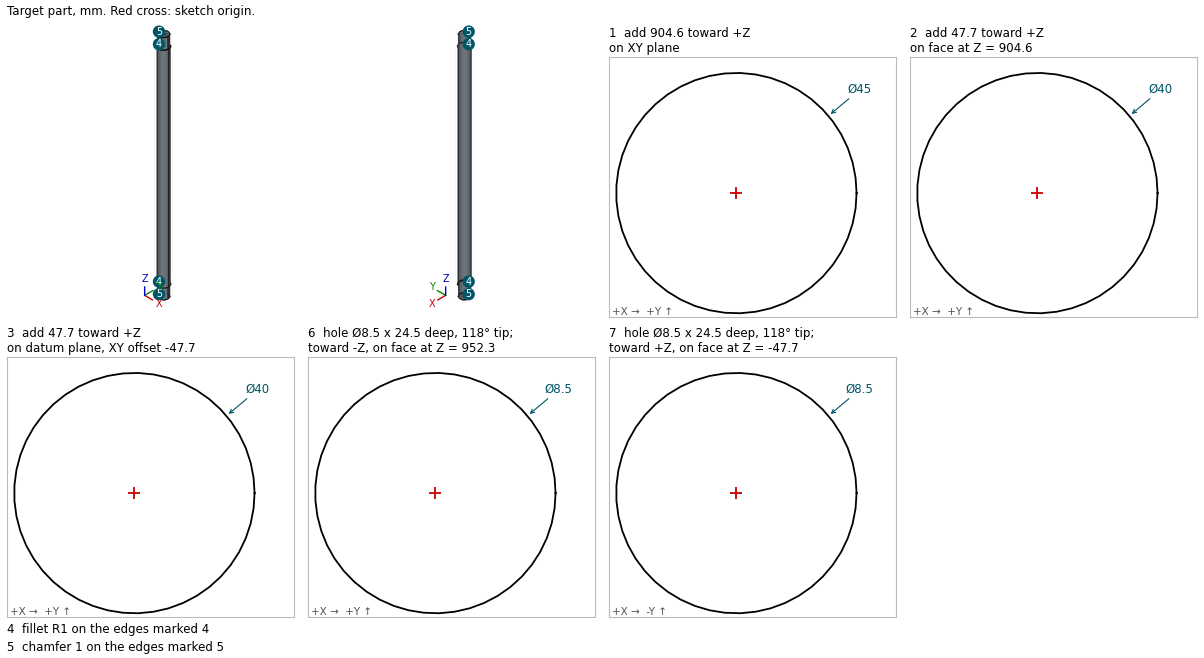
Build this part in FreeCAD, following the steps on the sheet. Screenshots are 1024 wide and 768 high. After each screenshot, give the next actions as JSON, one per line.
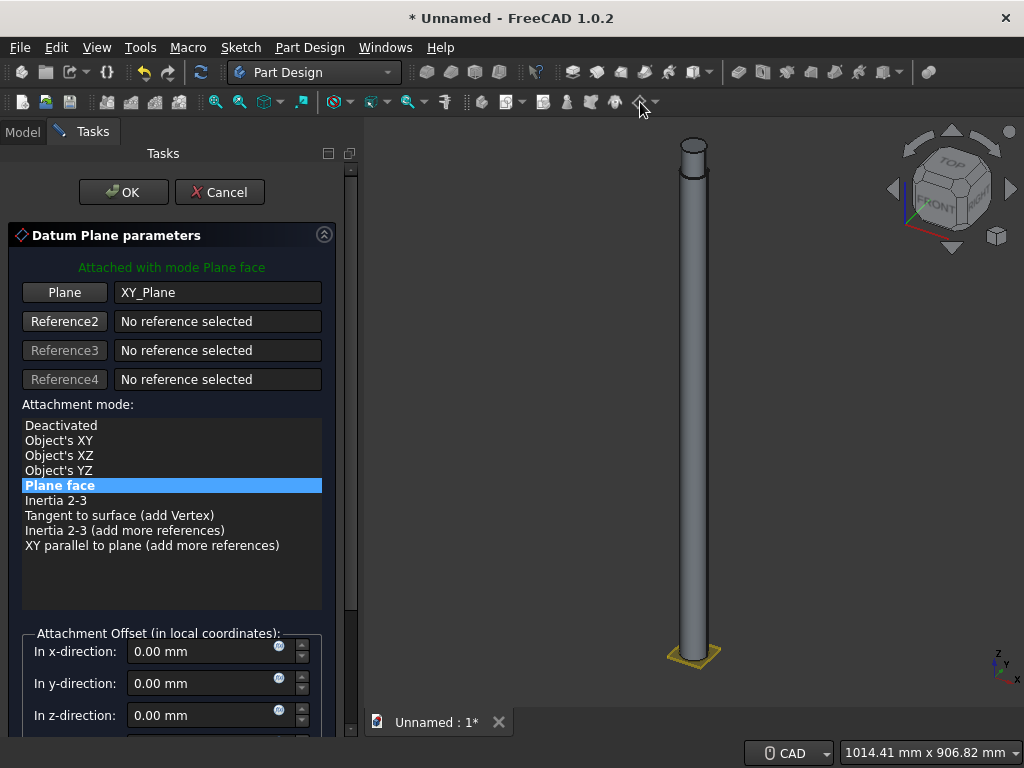
{"action": "triple_click", "coordinate": [210, 715]}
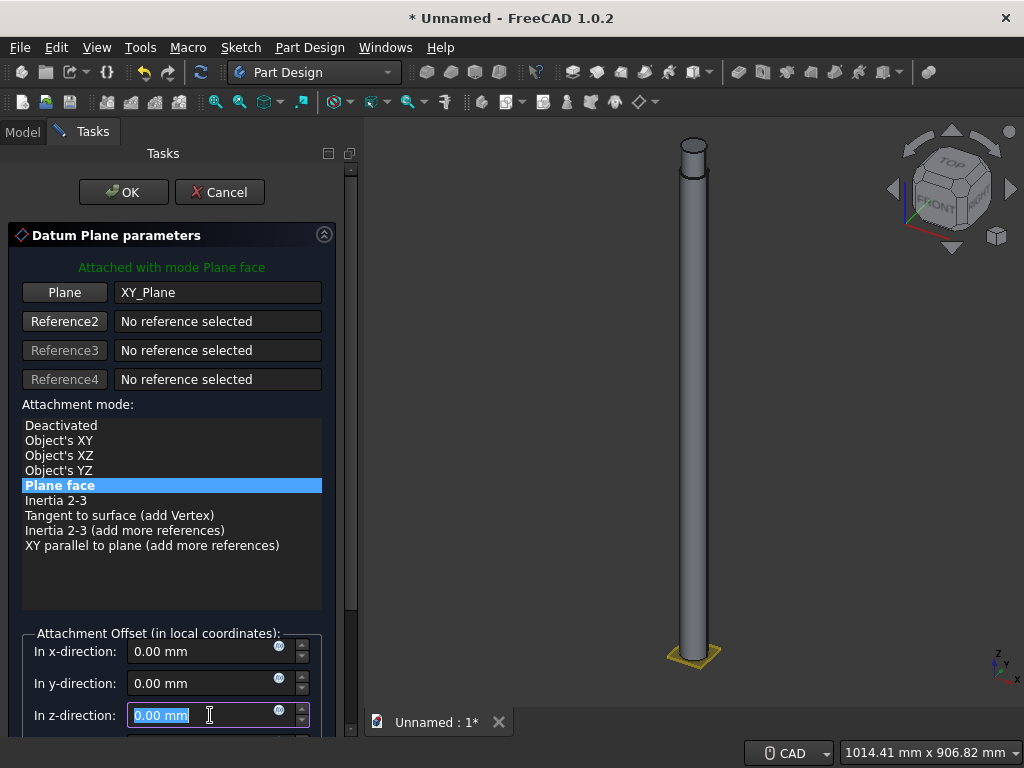
{"action": "type", "text": "-47.7"}
{"action": "key", "text": "Tab"}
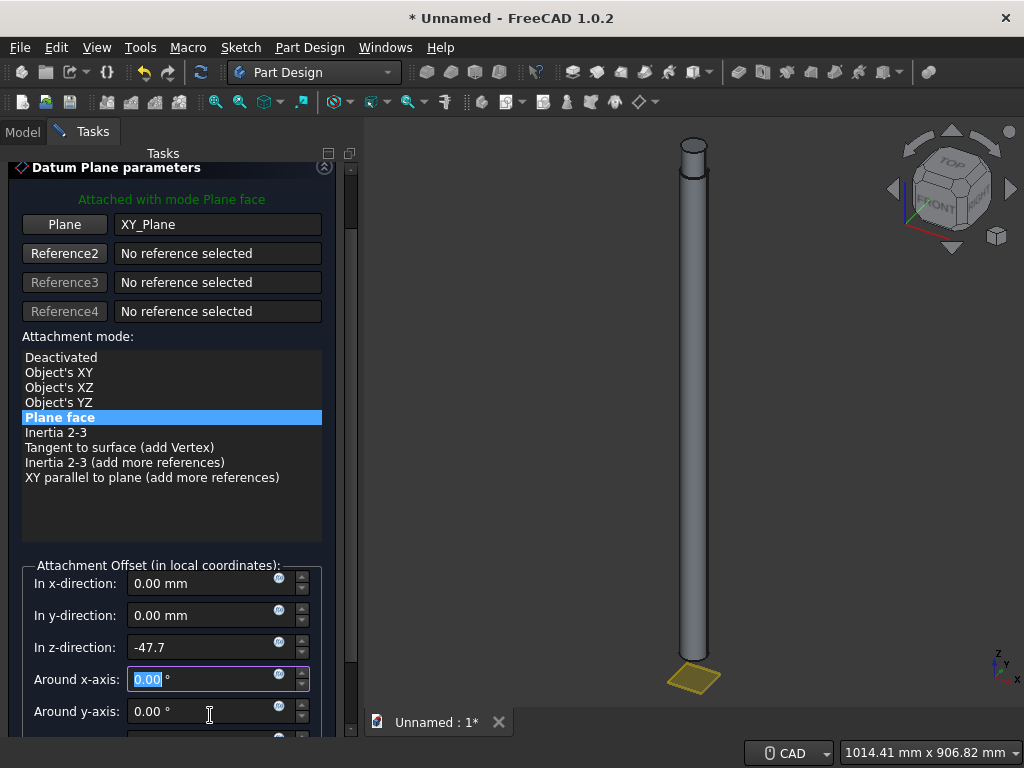
{"action": "scroll", "coordinate": [351, 450], "scroll_direction": "up", "scroll_amount": 2}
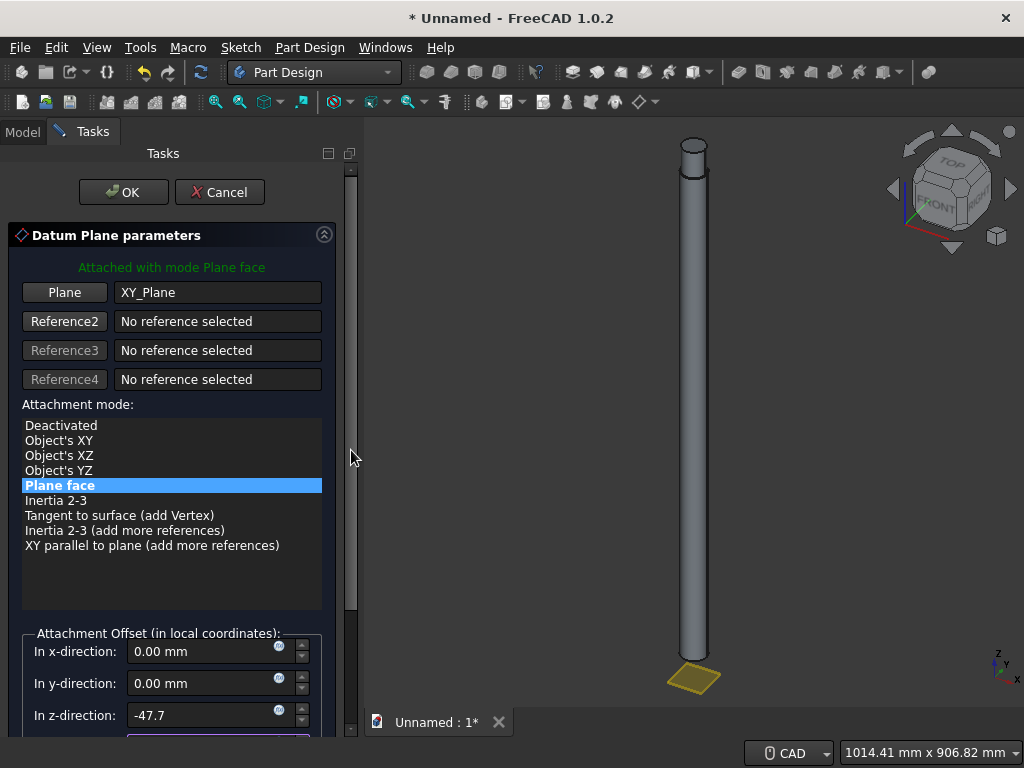
{"action": "left_click", "coordinate": [124, 192]}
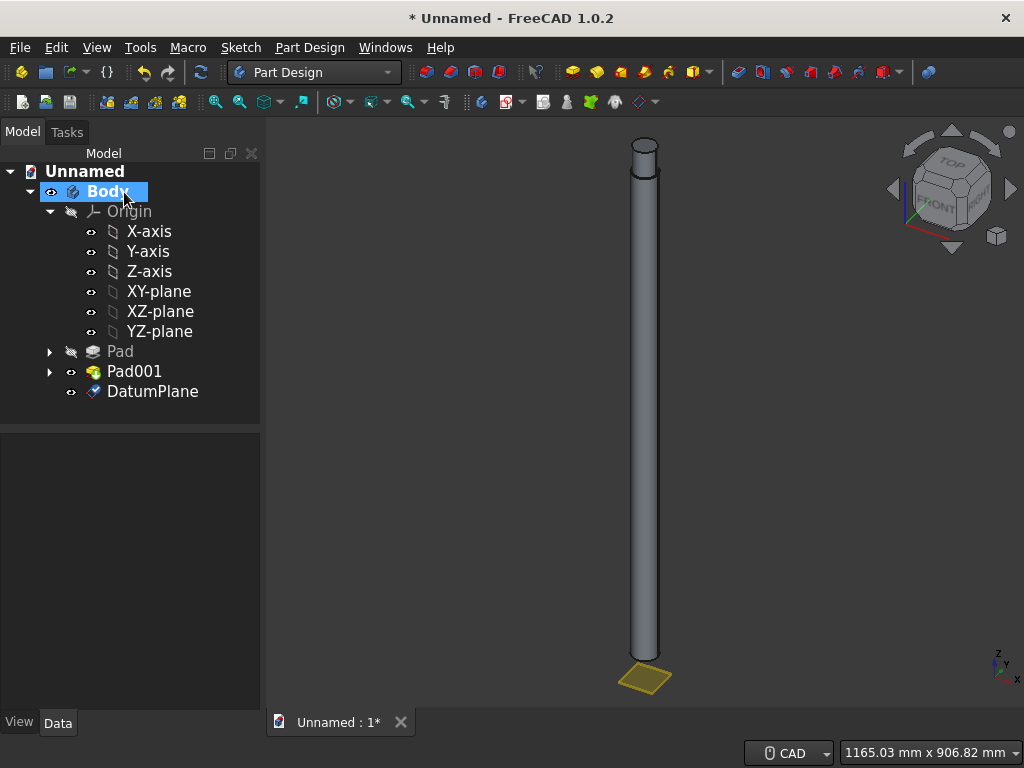
{"action": "left_click", "coordinate": [116, 392]}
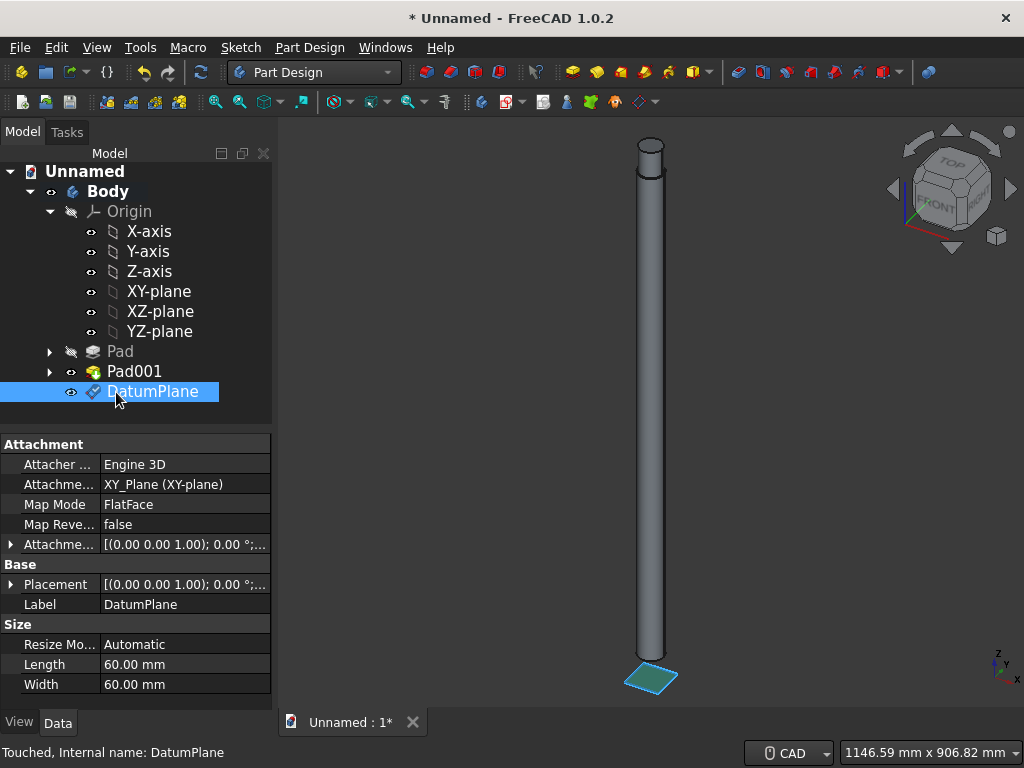
{"action": "left_click", "coordinate": [506, 102]}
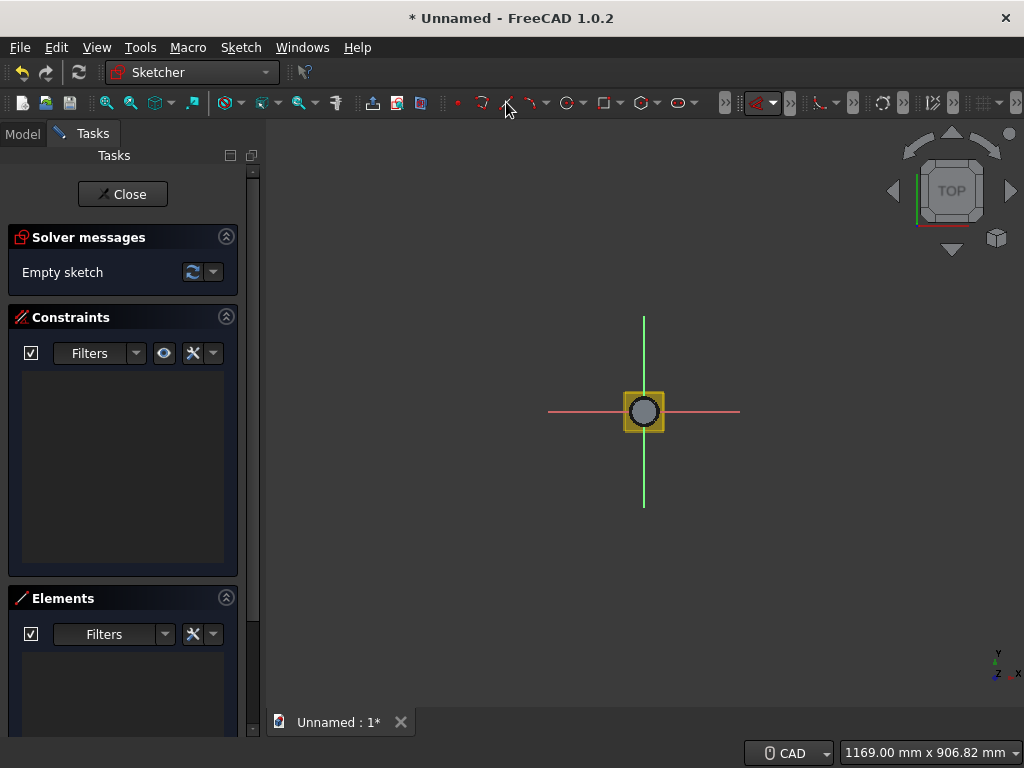
{"action": "left_click", "coordinate": [422, 104]}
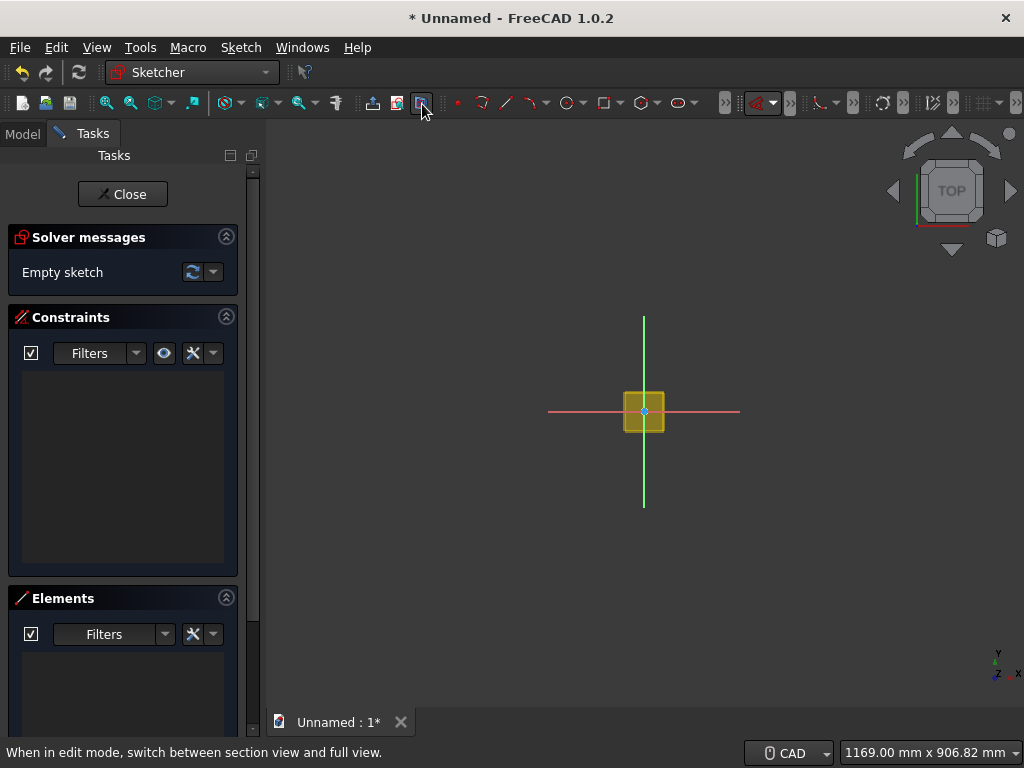
{"action": "scroll", "coordinate": [650, 412], "scroll_direction": "up", "scroll_amount": 13}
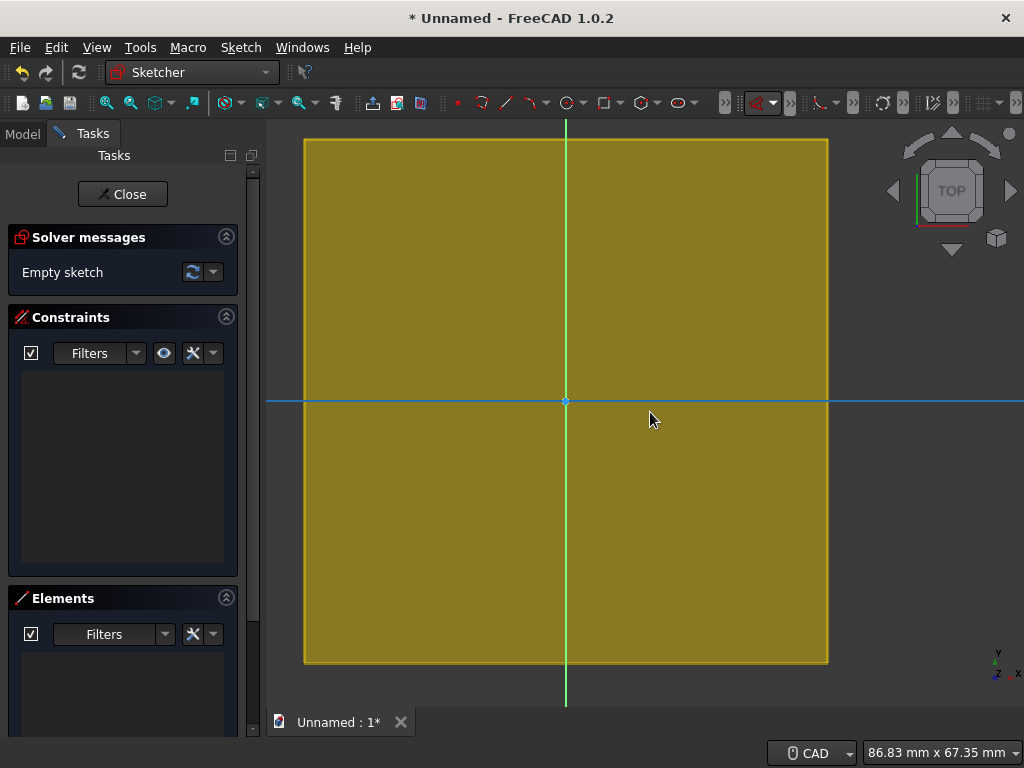
{"action": "left_click", "coordinate": [568, 104]}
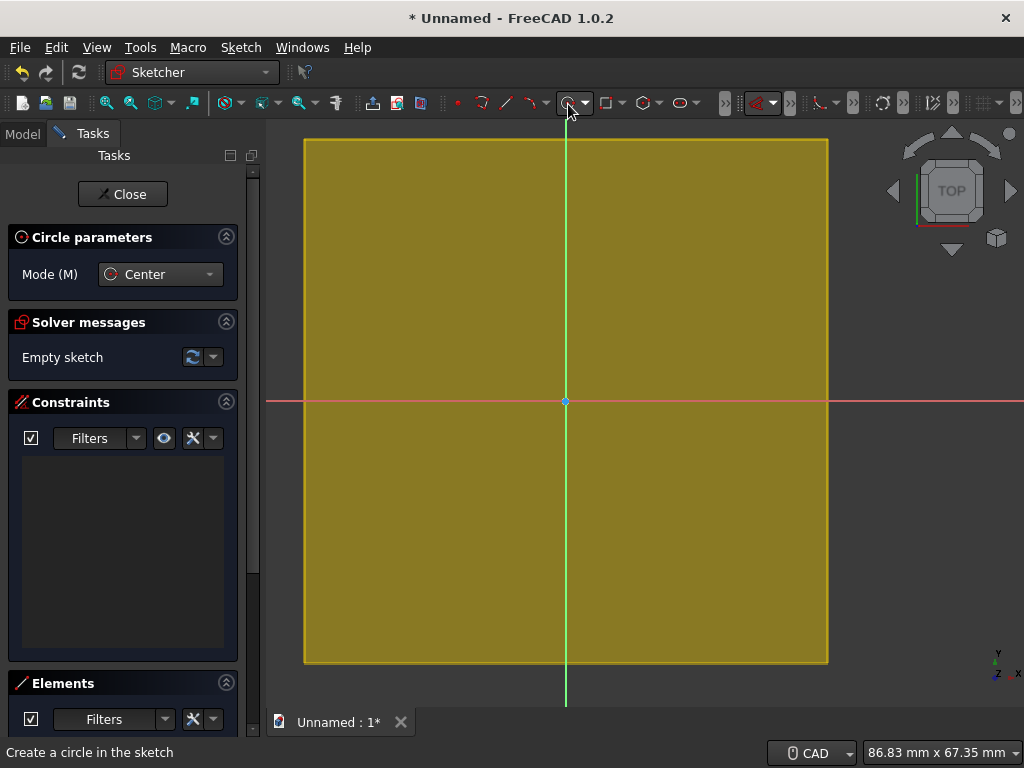
{"action": "left_click", "coordinate": [566, 401]}
{"action": "mouse_move", "coordinate": [689, 278]}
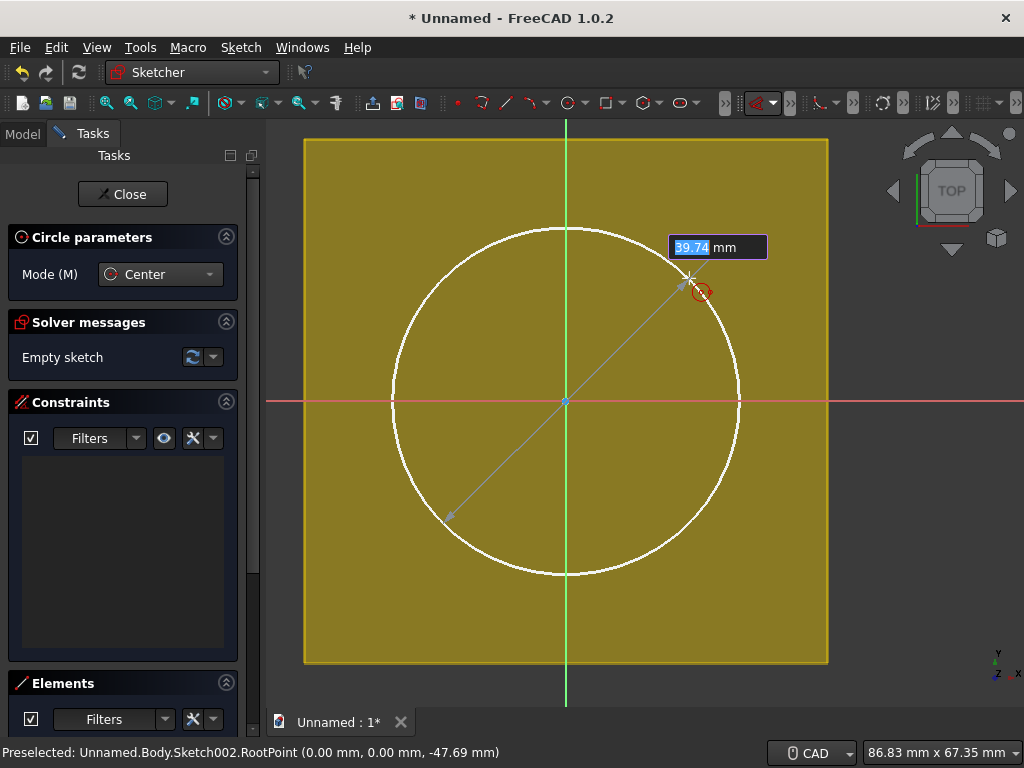
{"action": "type", "text": "40"}
{"action": "key", "text": "Return"}
{"action": "key", "text": "Escape"}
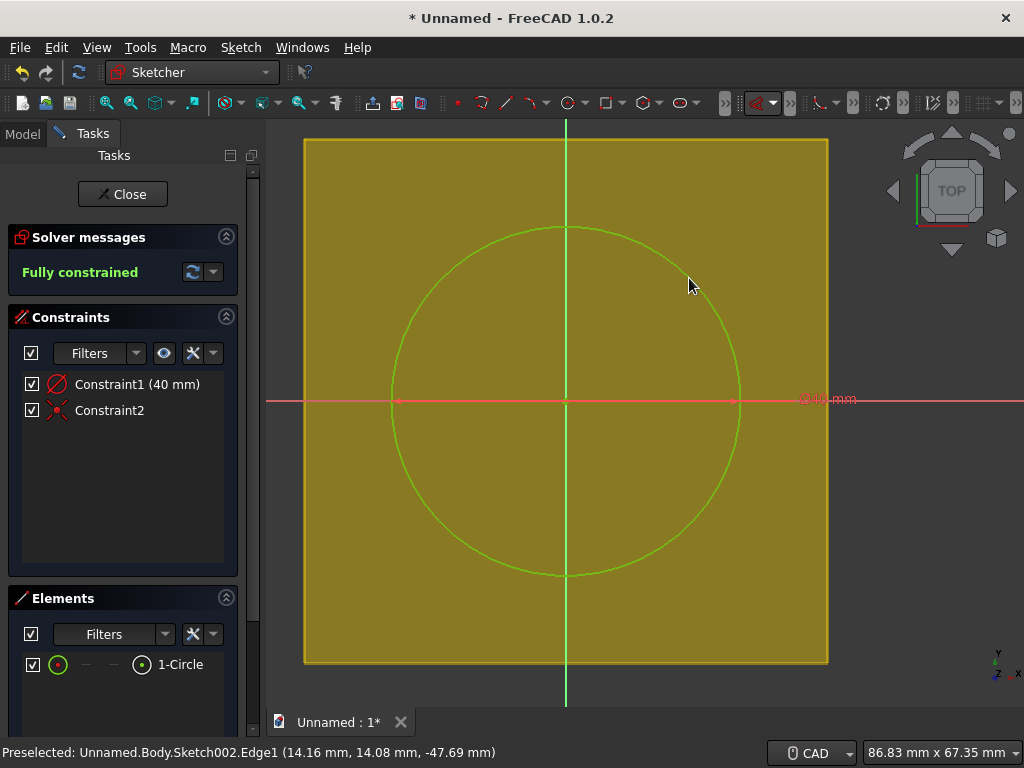
{"action": "left_click", "coordinate": [123, 194]}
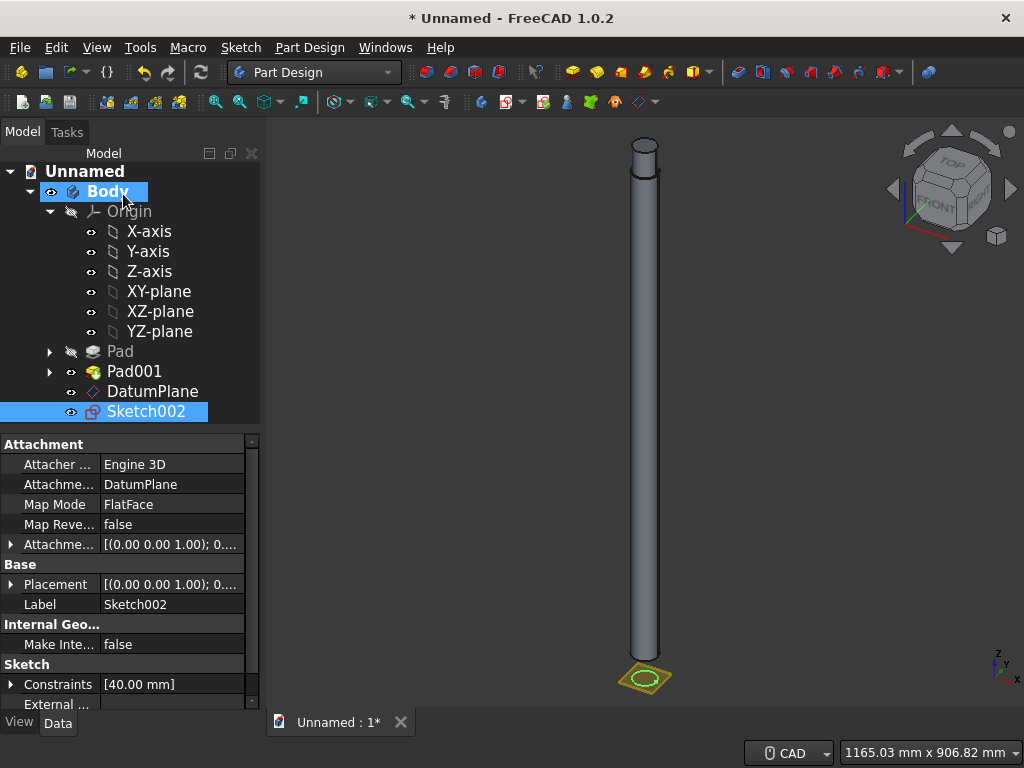
{"action": "left_click", "coordinate": [574, 72]}